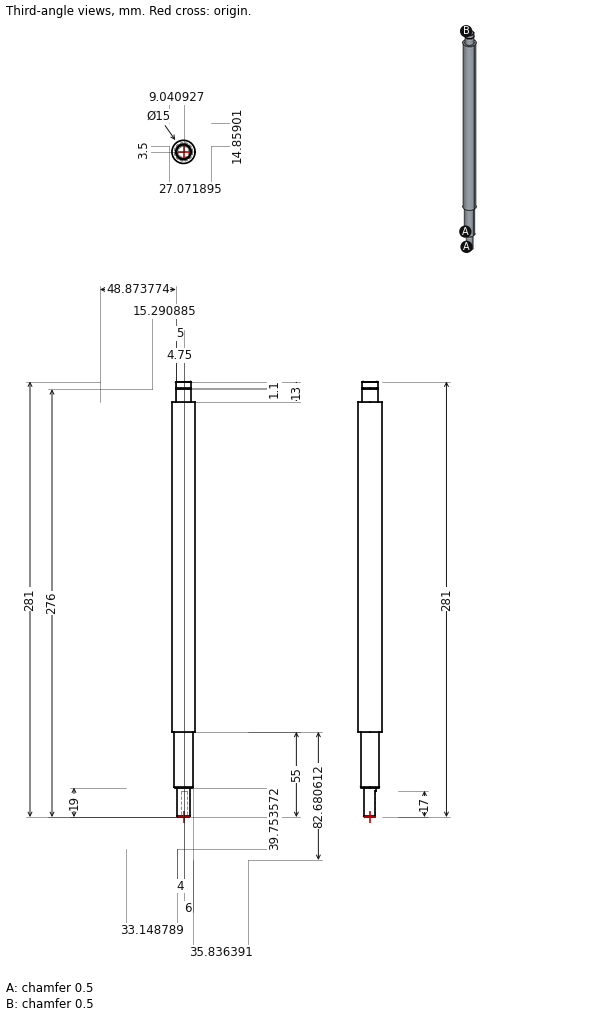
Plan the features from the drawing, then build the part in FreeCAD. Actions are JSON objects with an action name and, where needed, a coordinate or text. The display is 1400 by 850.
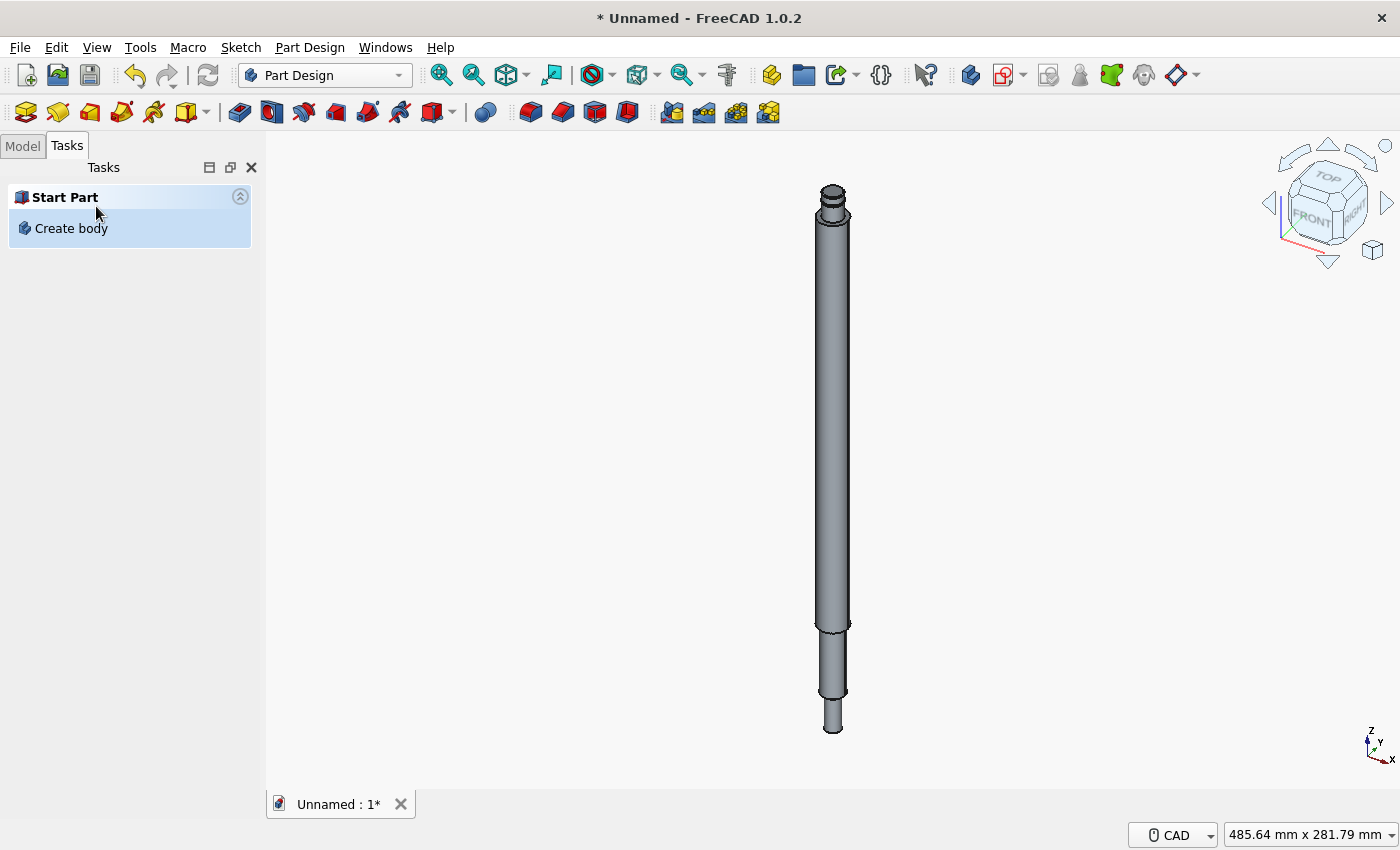
{"action": "key", "text": "5"}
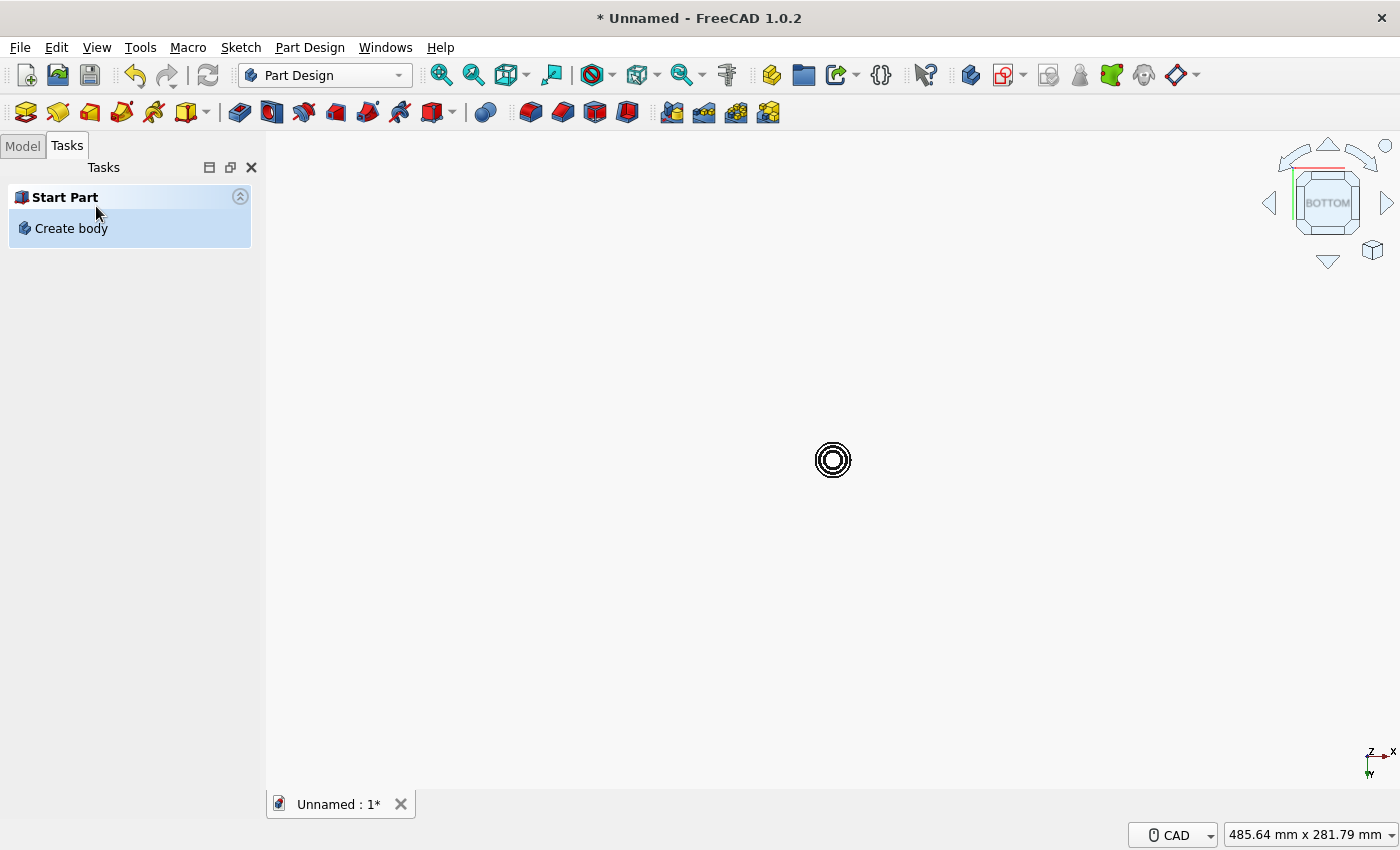
{"action": "left_click", "coordinate": [442, 76]}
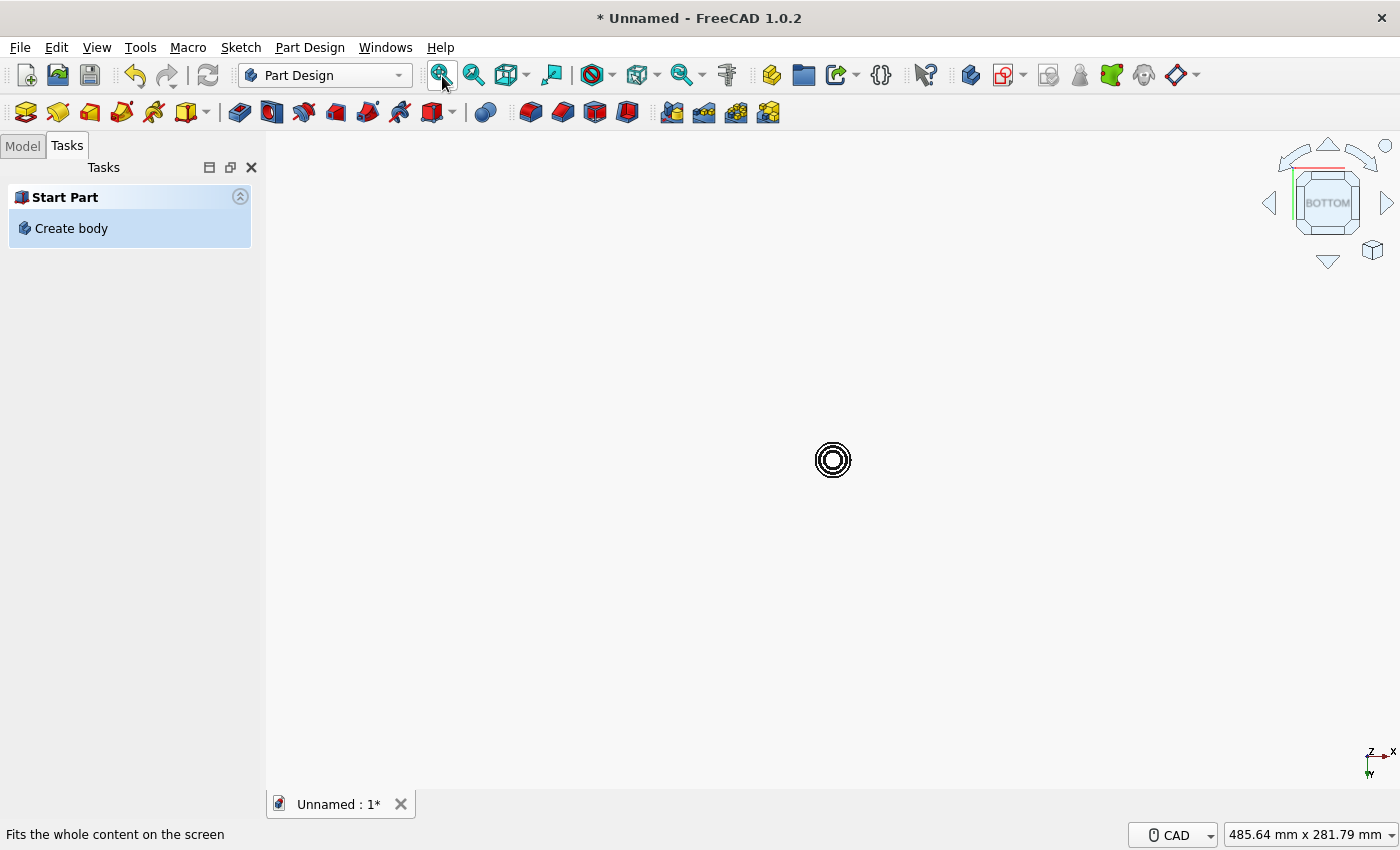
{"action": "key", "text": "1"}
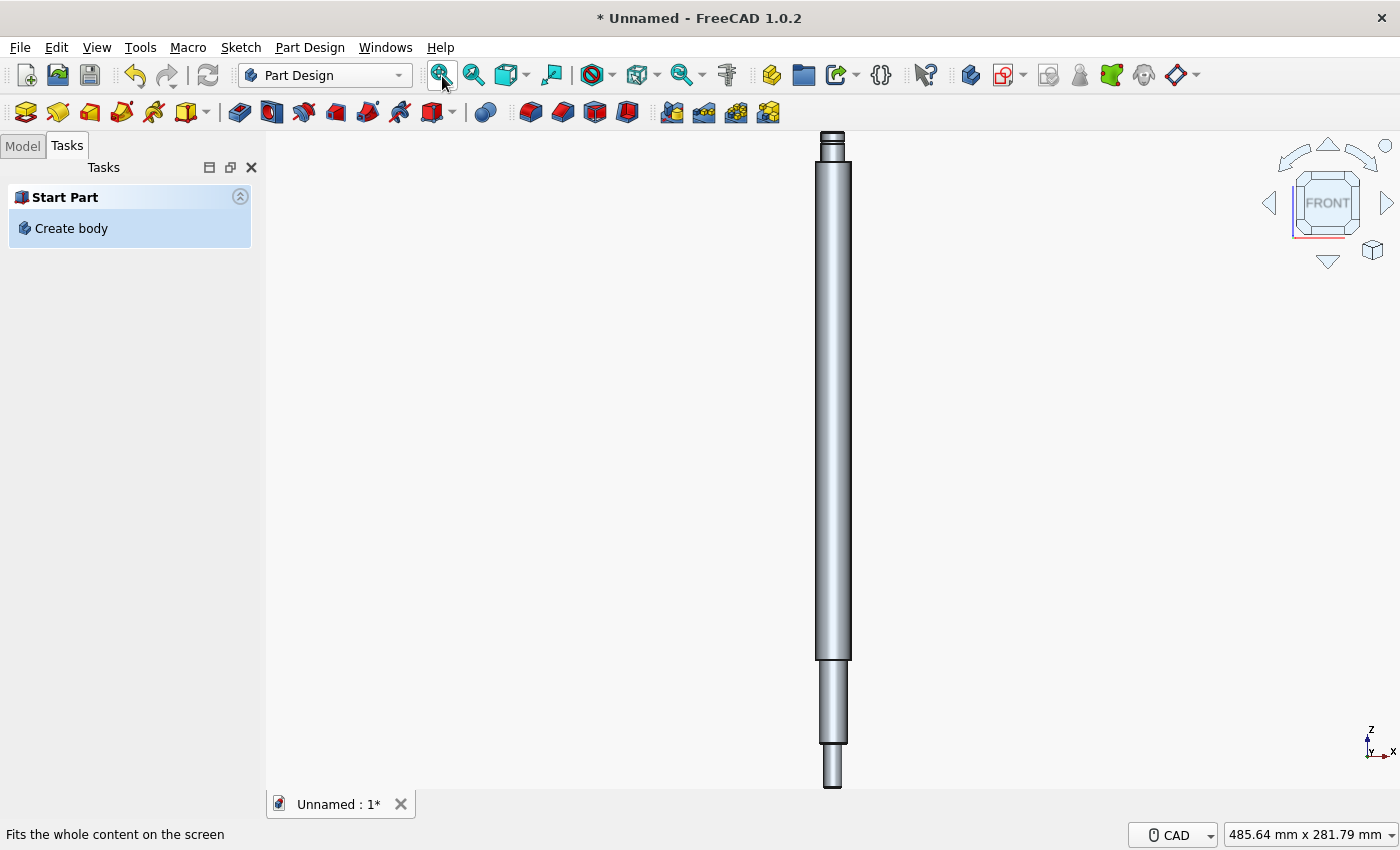
{"action": "key", "text": "3"}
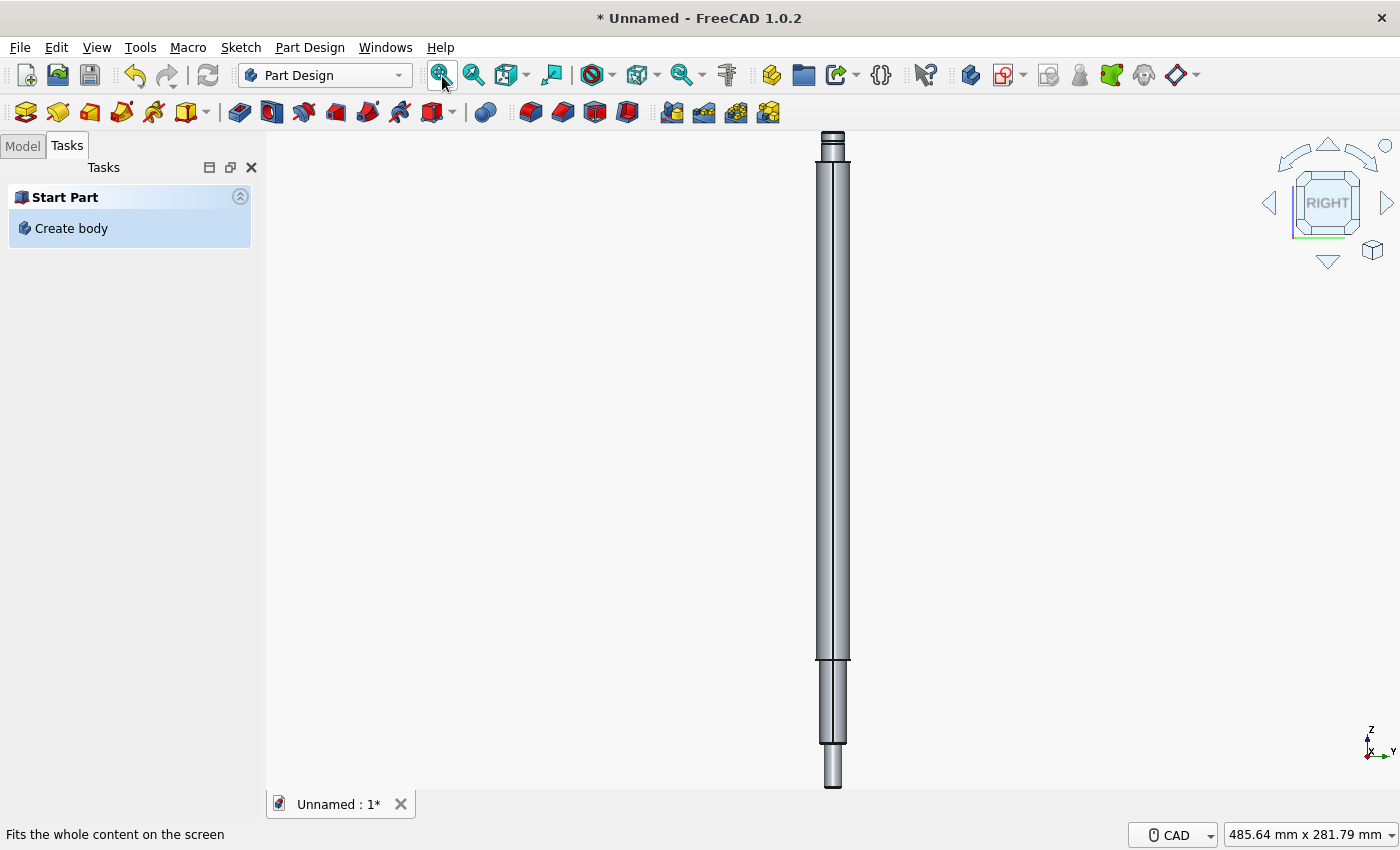
{"action": "left_click", "coordinate": [1004, 76]}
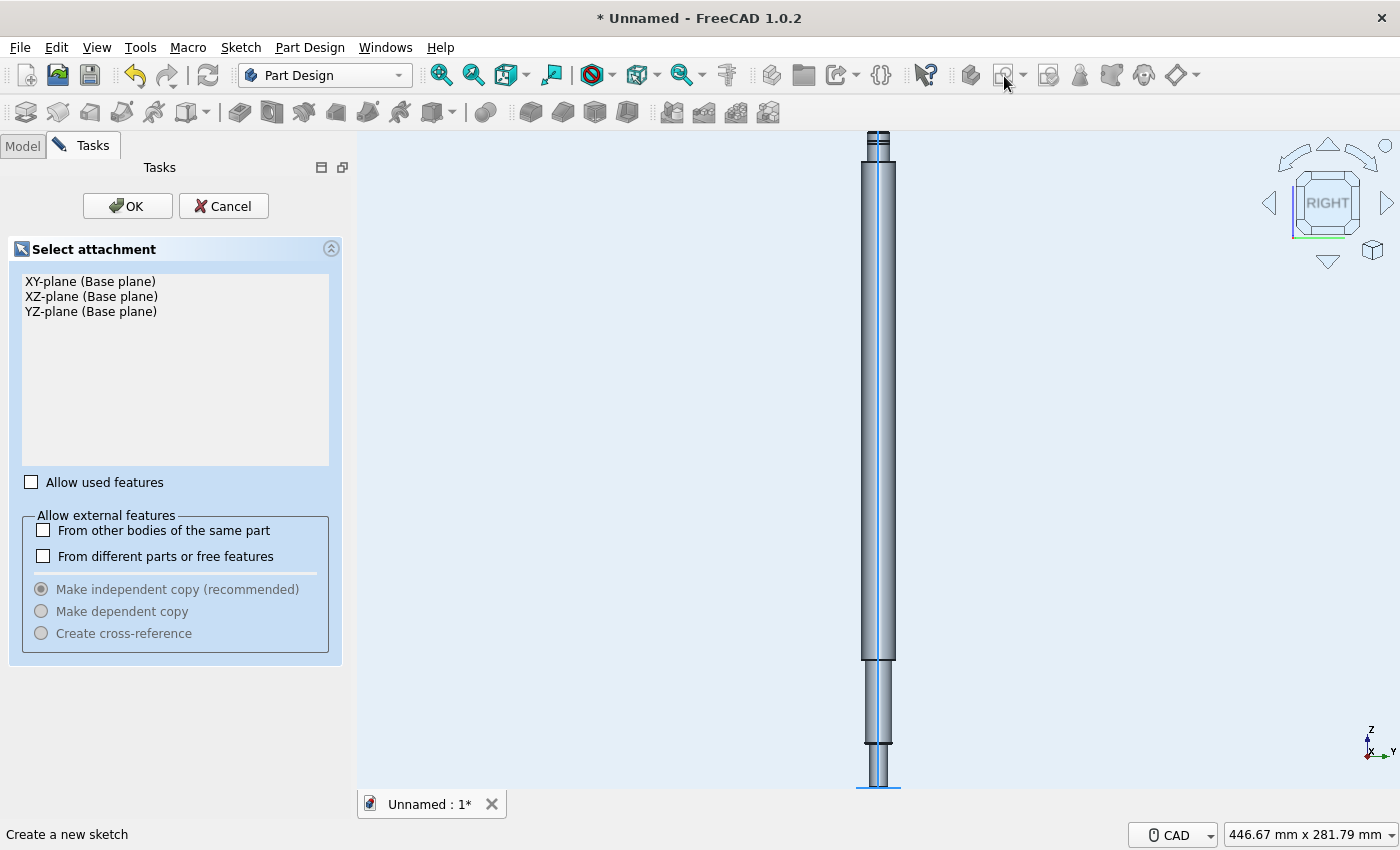
{"action": "left_click", "coordinate": [82, 282]}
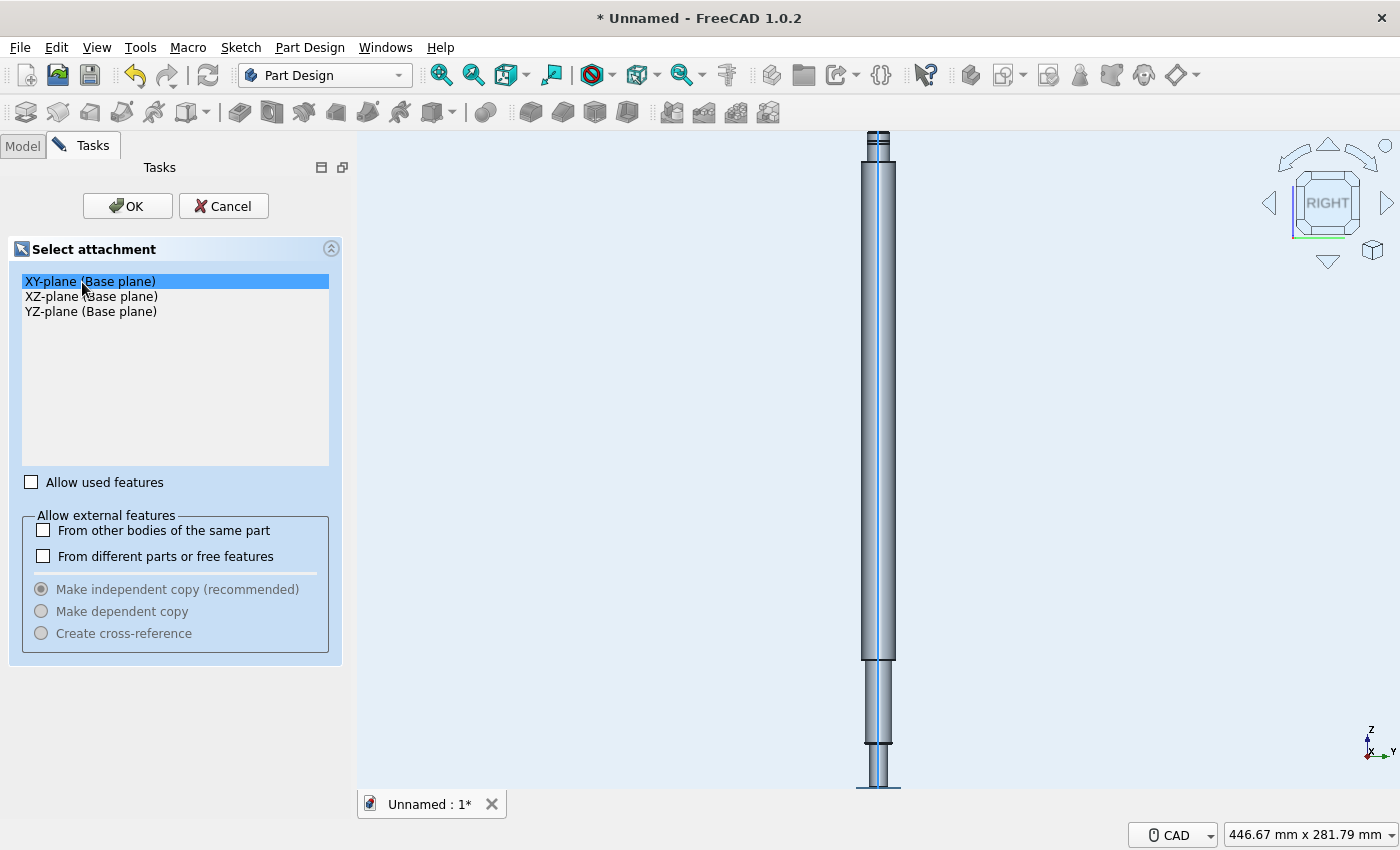
{"action": "left_click", "coordinate": [128, 206]}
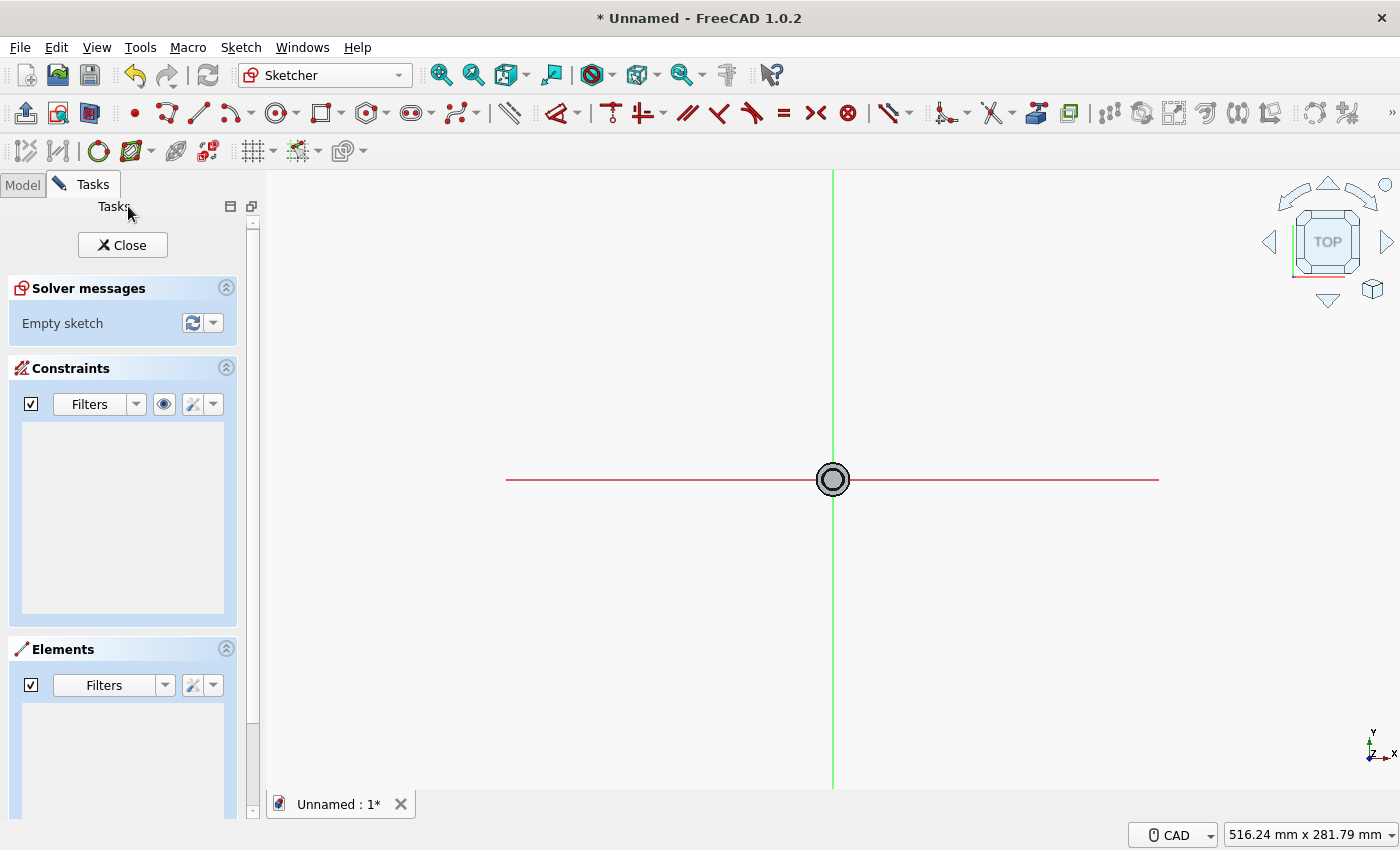
{"action": "left_click", "coordinate": [90, 114]}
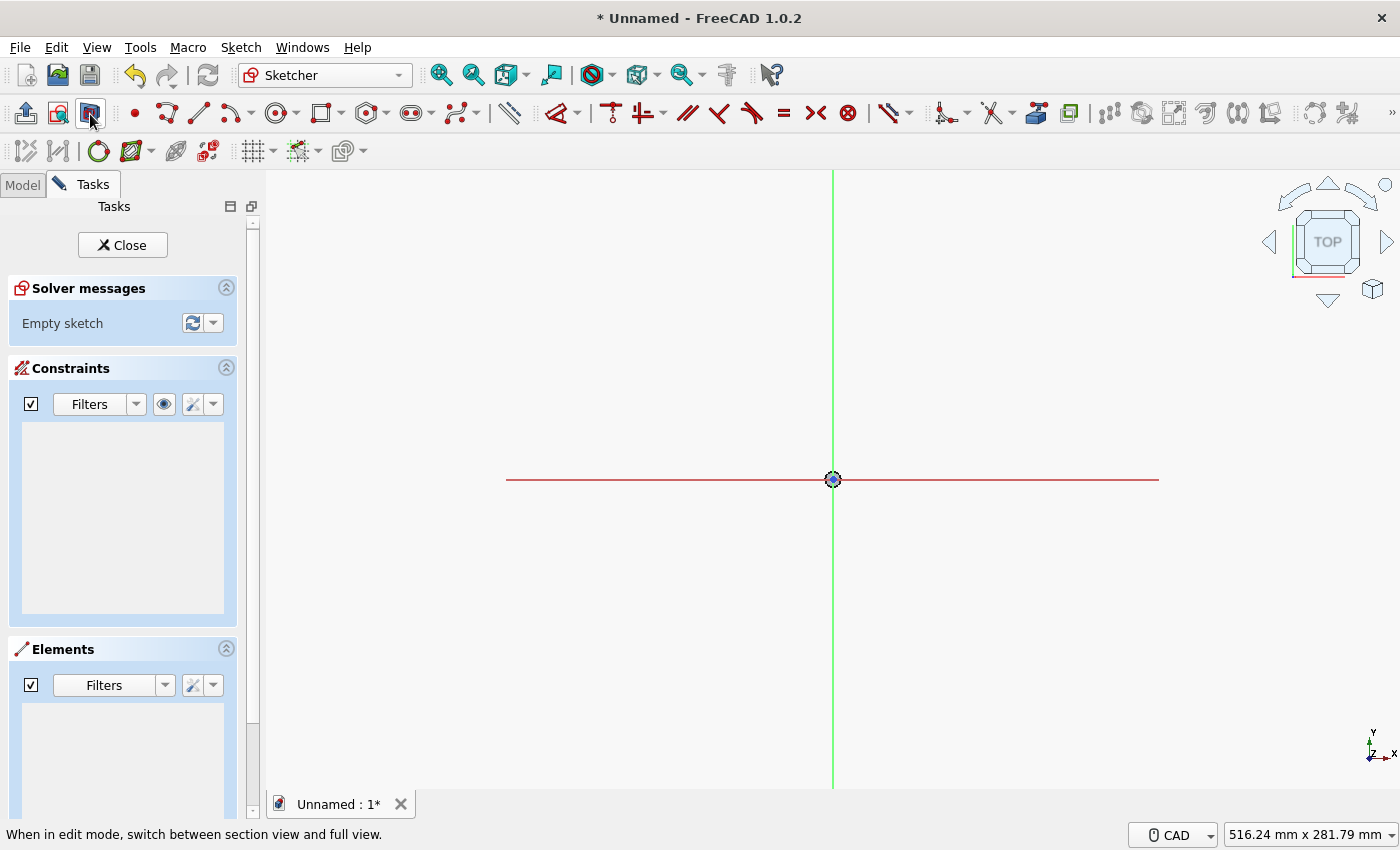
{"action": "scroll", "coordinate": [853, 457], "scroll_direction": "up", "scroll_amount": 11}